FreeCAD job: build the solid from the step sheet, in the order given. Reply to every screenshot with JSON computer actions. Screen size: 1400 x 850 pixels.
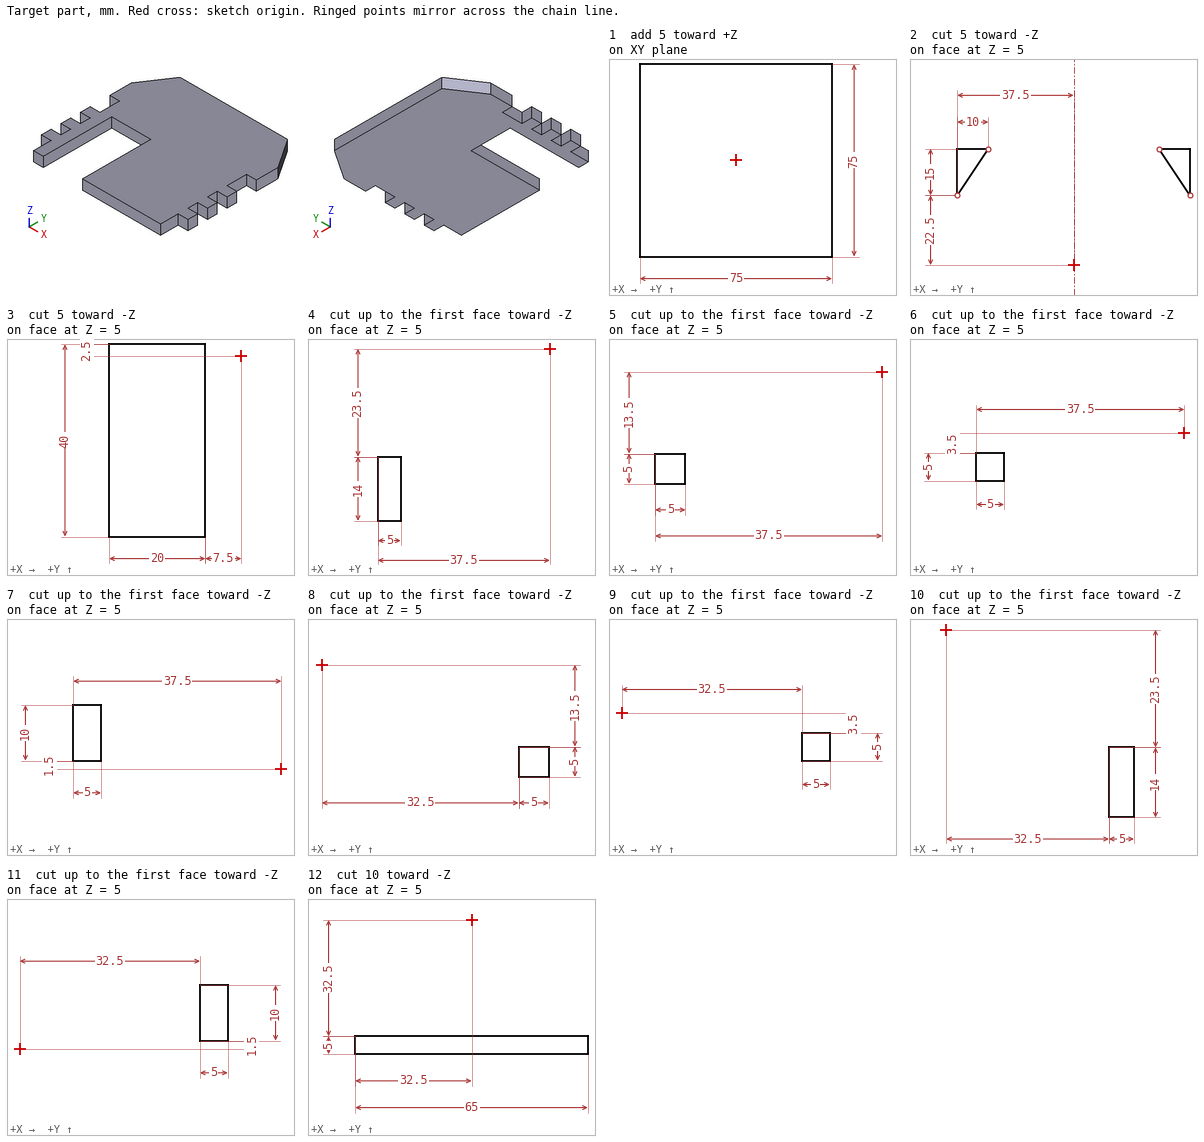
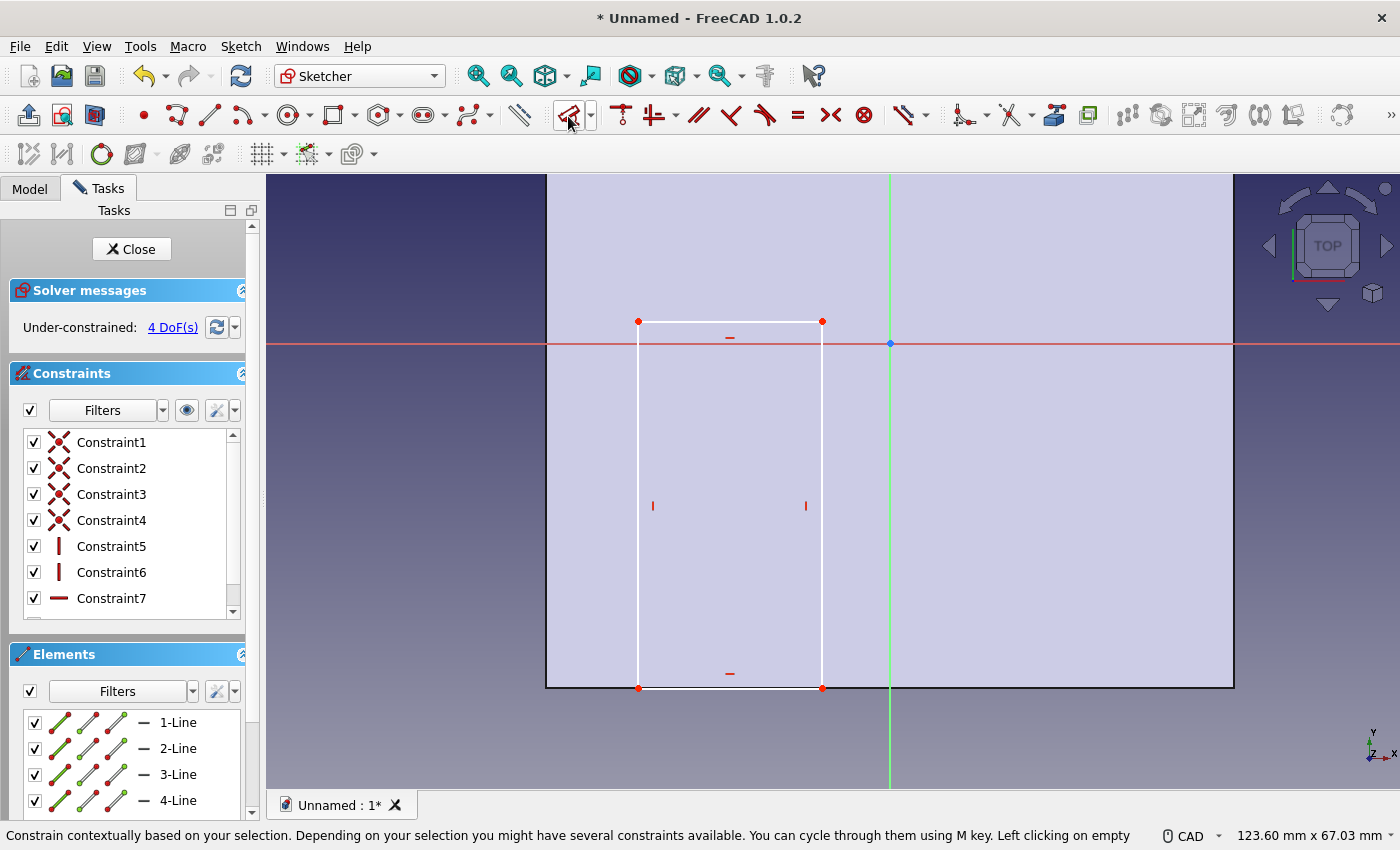
{"action": "left_click", "coordinate": [638, 432]}
{"action": "left_click", "coordinate": [604, 506]}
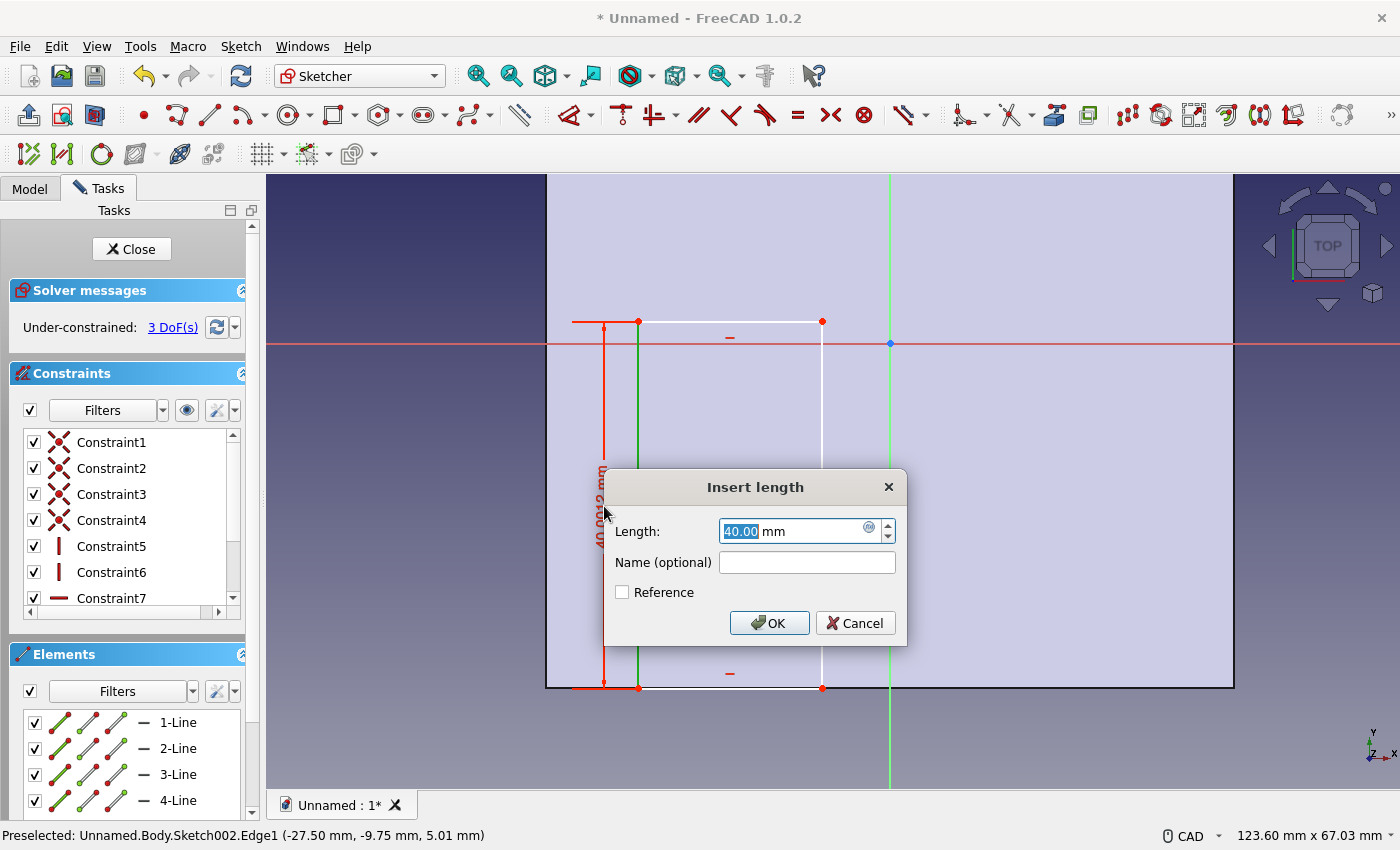
{"action": "type", "text": "40"}
{"action": "key", "text": "Return"}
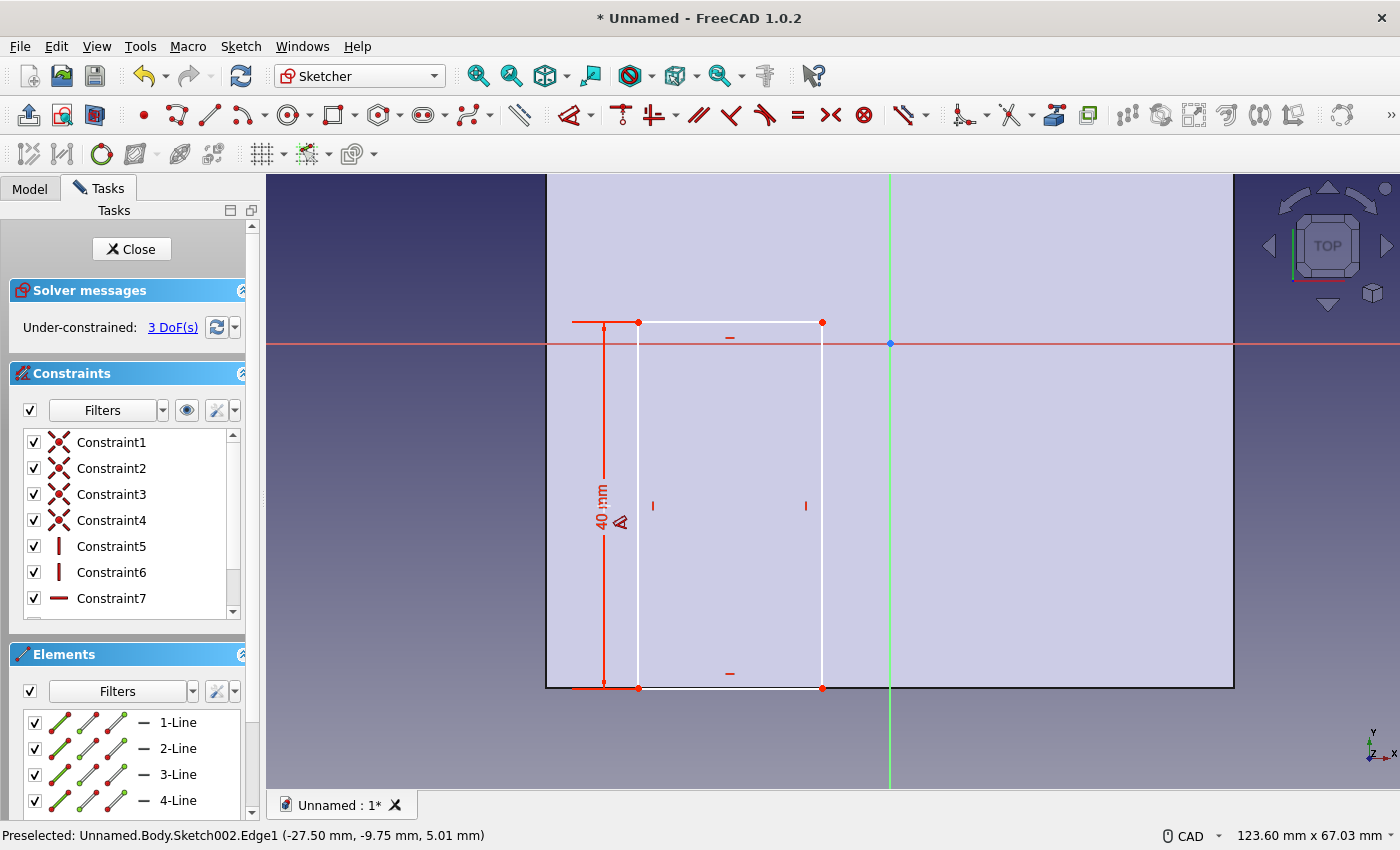
{"action": "left_click", "coordinate": [693, 689]}
{"action": "left_click", "coordinate": [730, 723]}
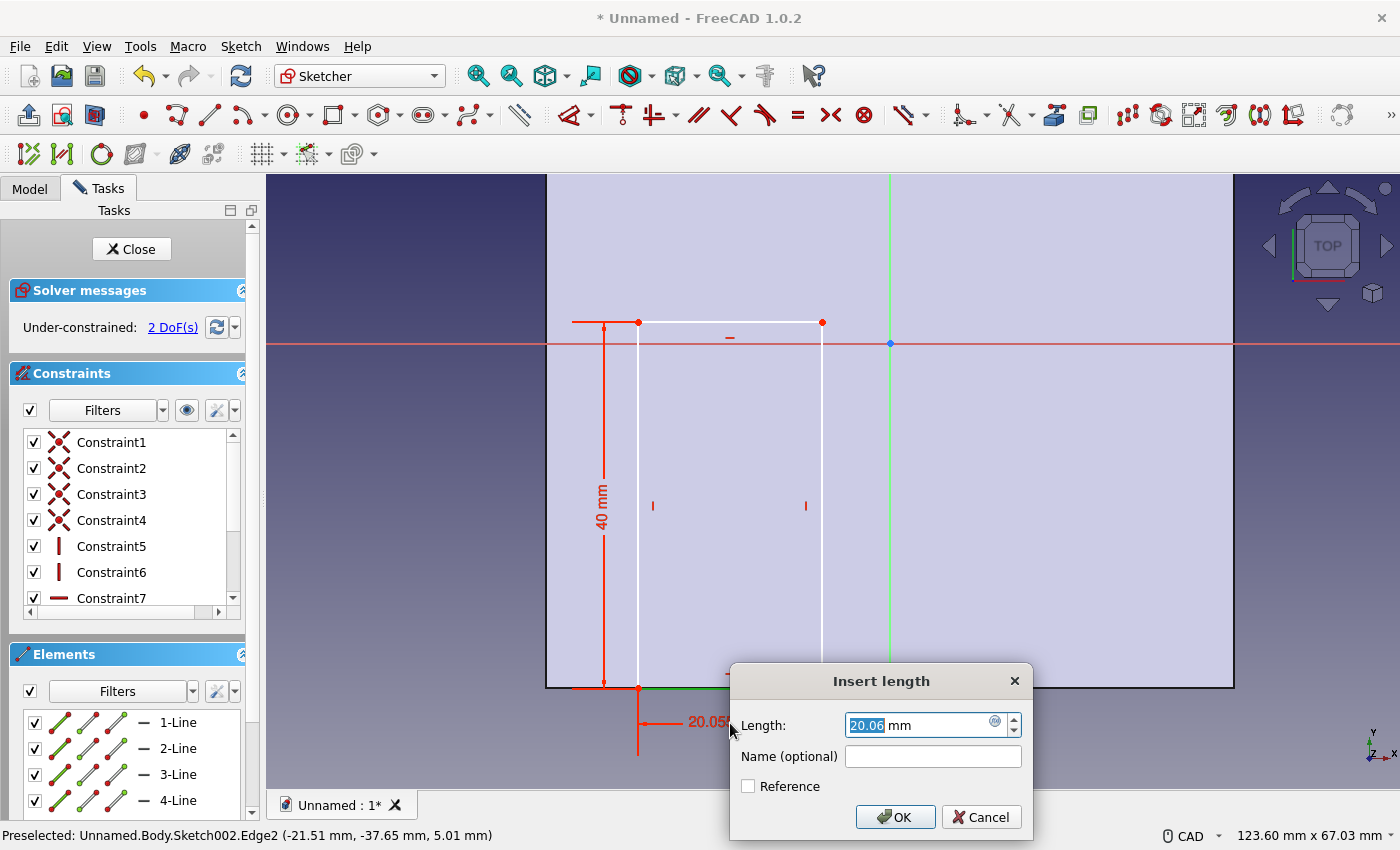
{"action": "type", "text": "20"}
{"action": "key", "text": "Return"}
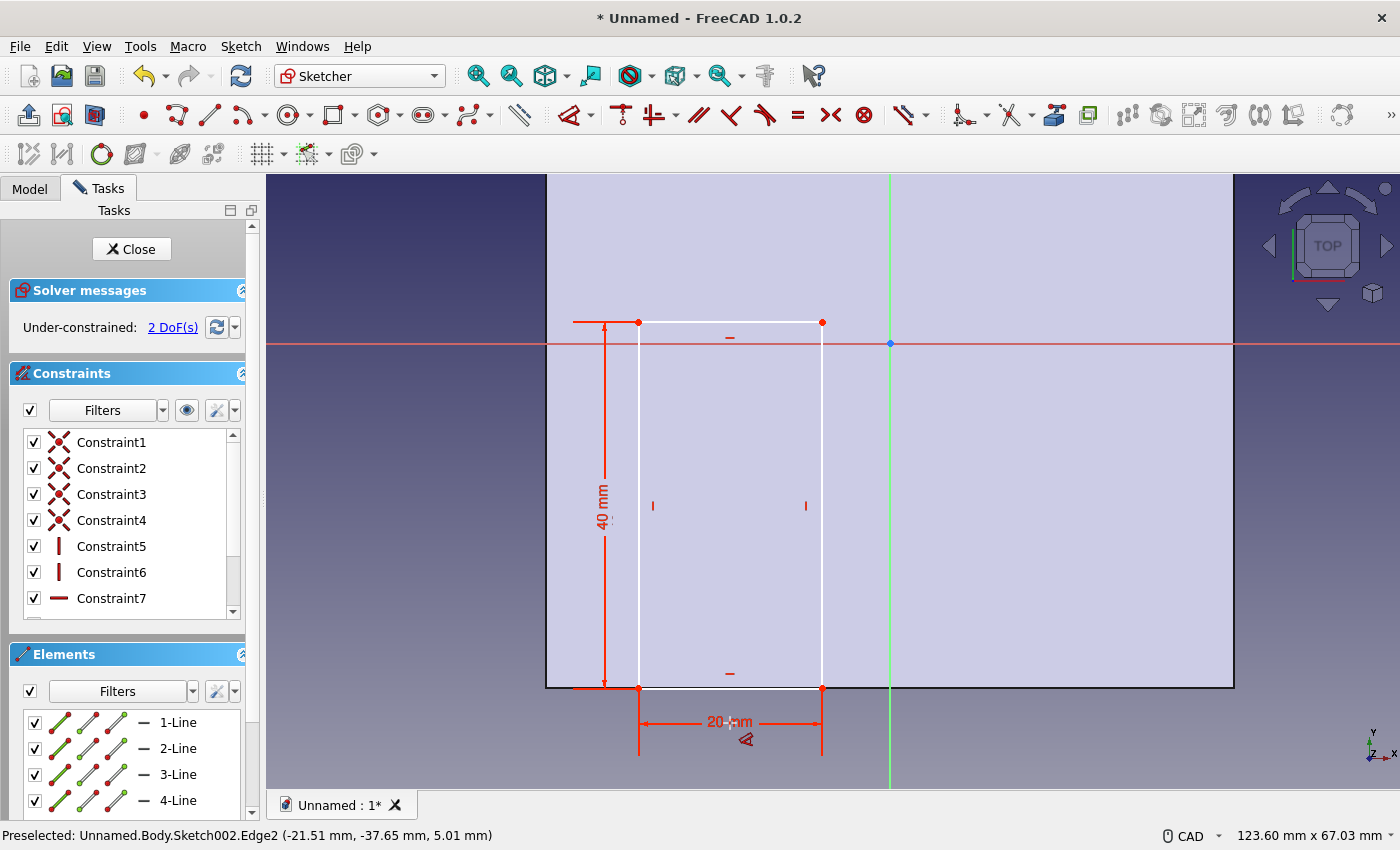
{"action": "scroll", "coordinate": [639, 322], "scroll_direction": "up", "scroll_amount": 3}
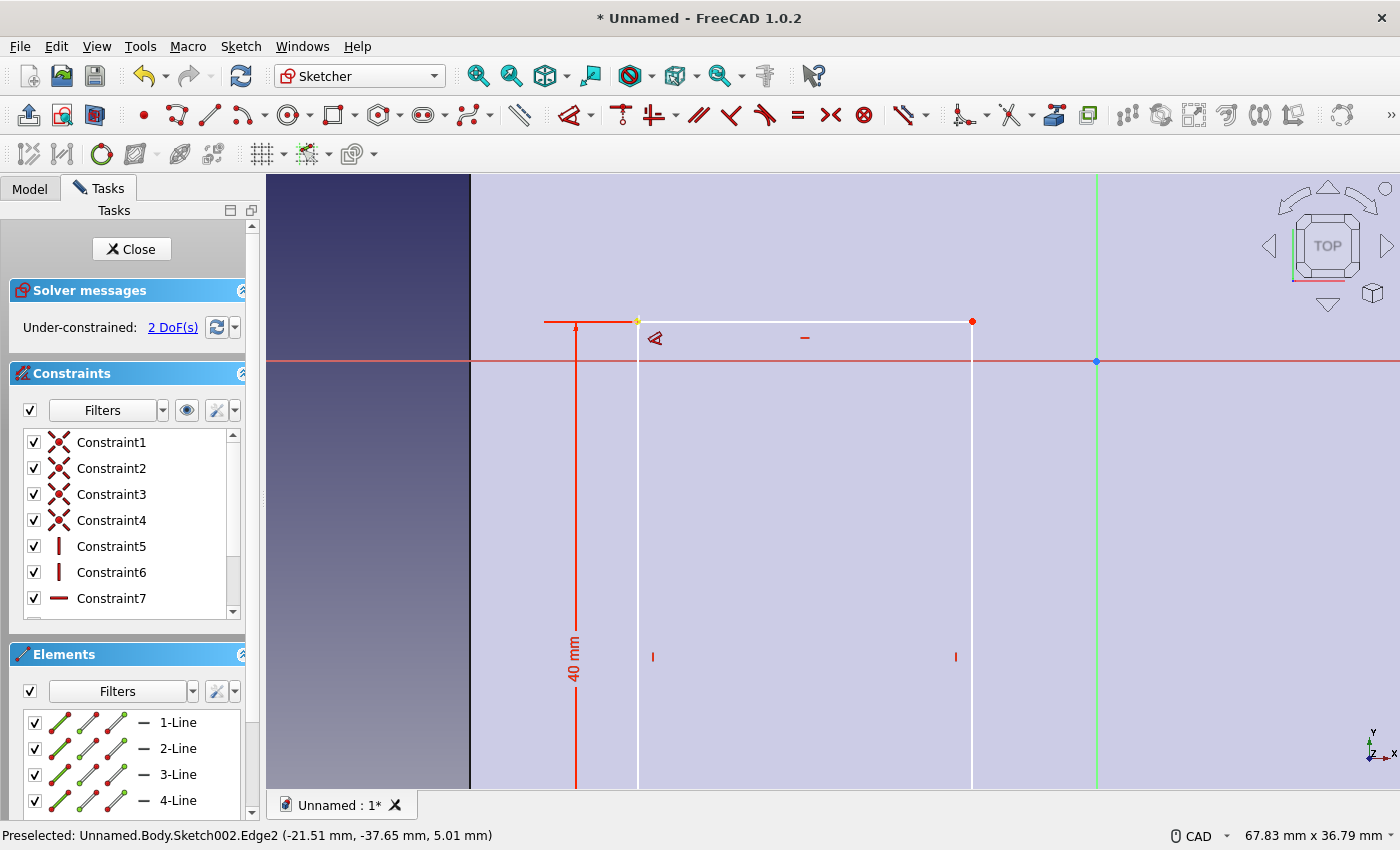
{"action": "left_click", "coordinate": [638, 322]}
{"action": "left_click", "coordinate": [1131, 341]}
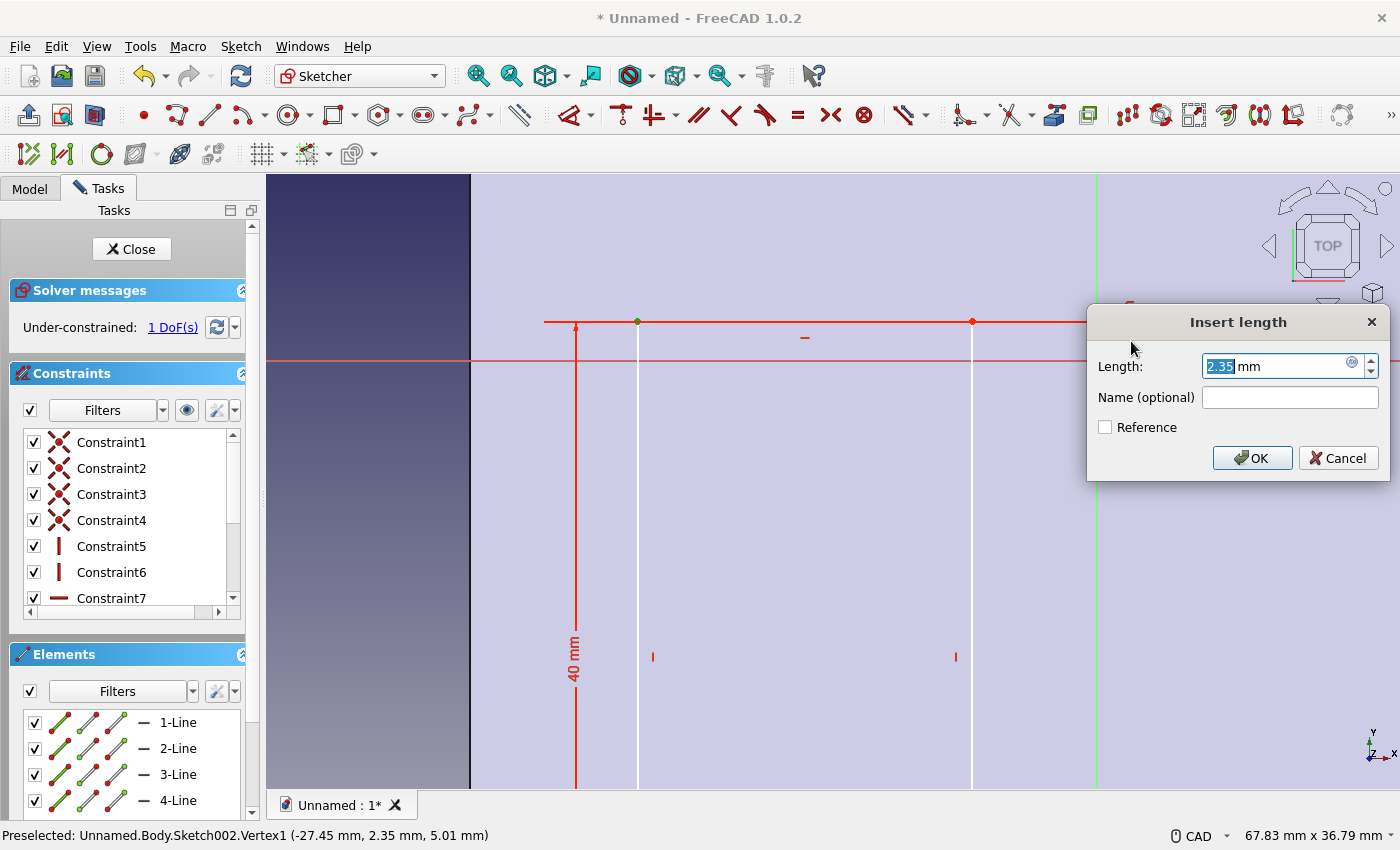
{"action": "type", "text": "2.5"}
{"action": "key", "text": "Return"}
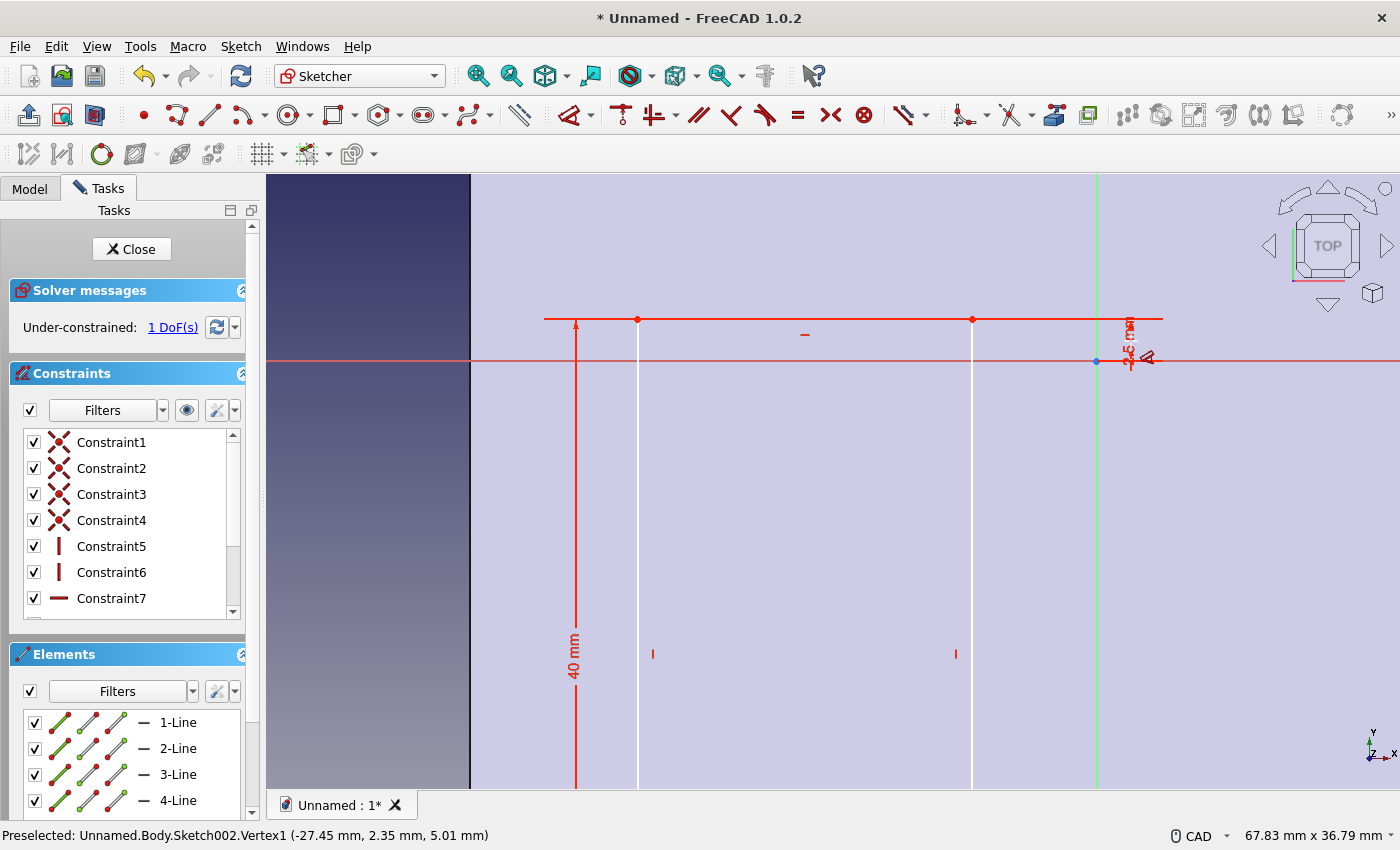
{"action": "scroll", "coordinate": [640, 272], "scroll_direction": "down", "scroll_amount": 3}